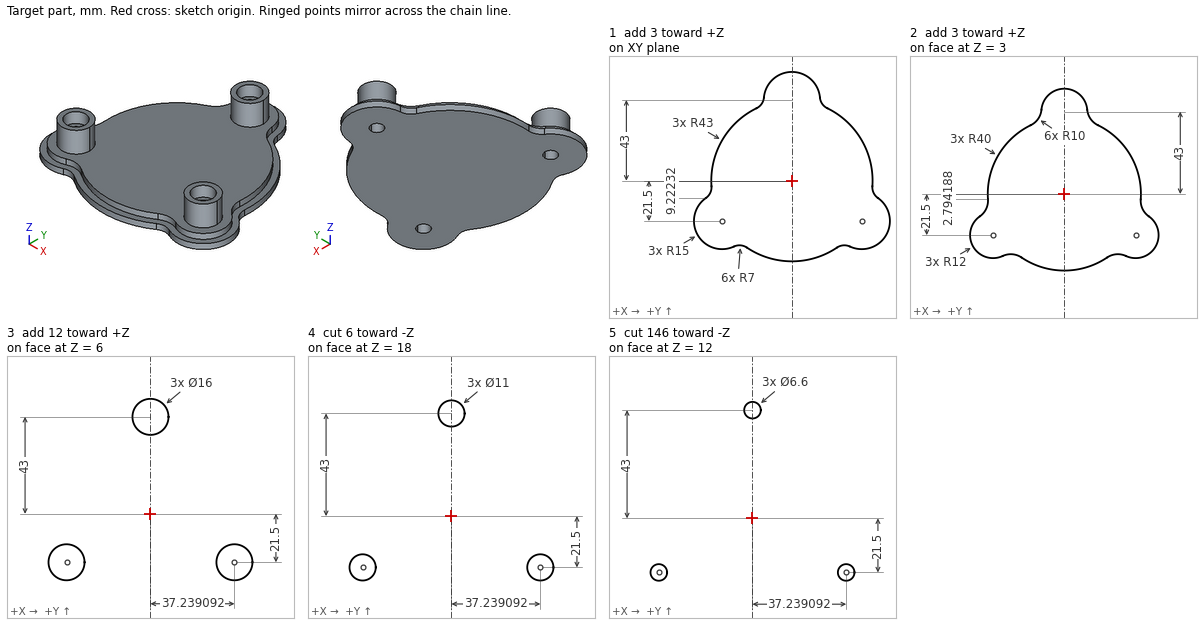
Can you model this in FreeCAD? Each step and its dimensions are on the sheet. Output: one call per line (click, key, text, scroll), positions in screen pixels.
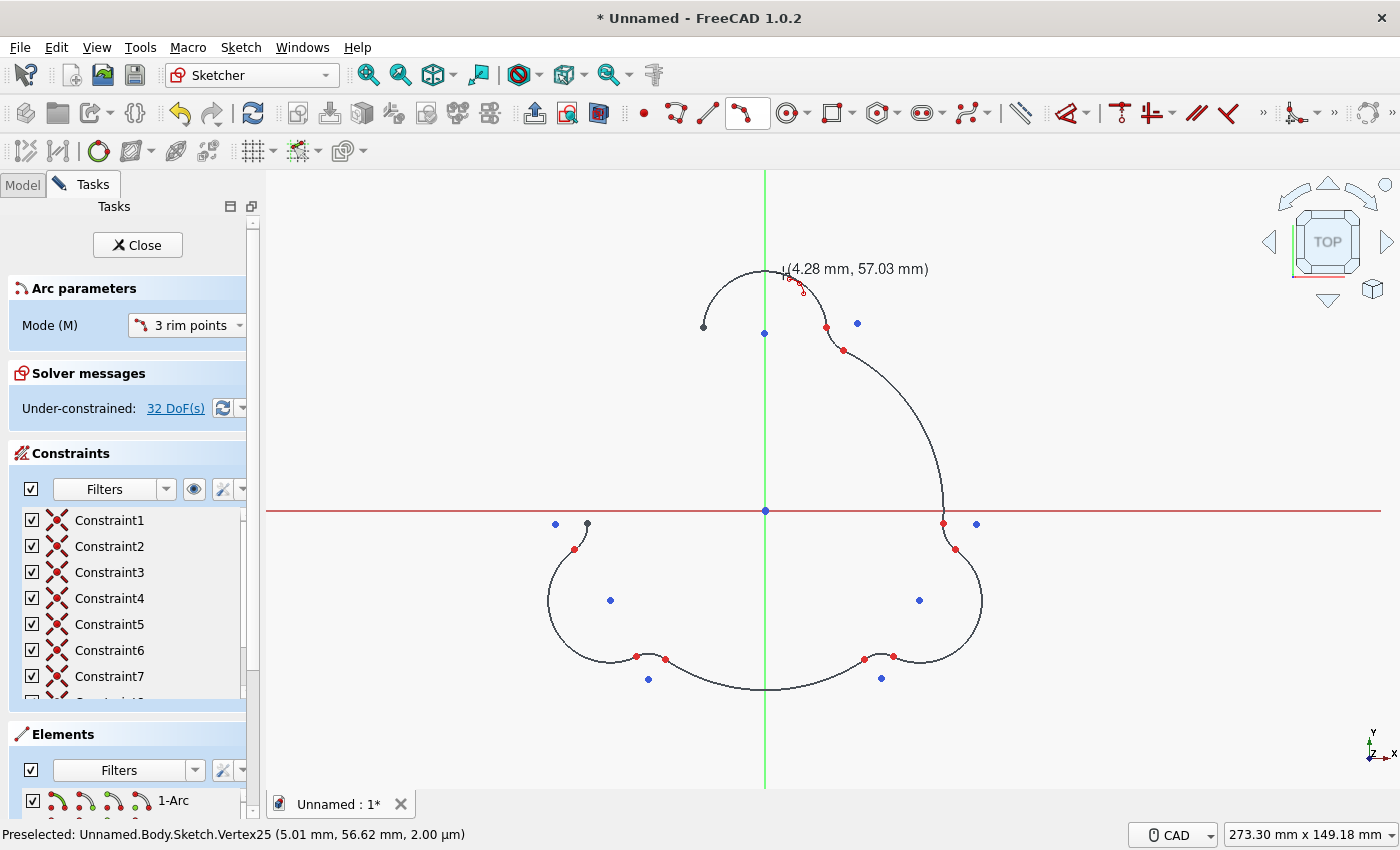
click(703, 328)
click(687, 350)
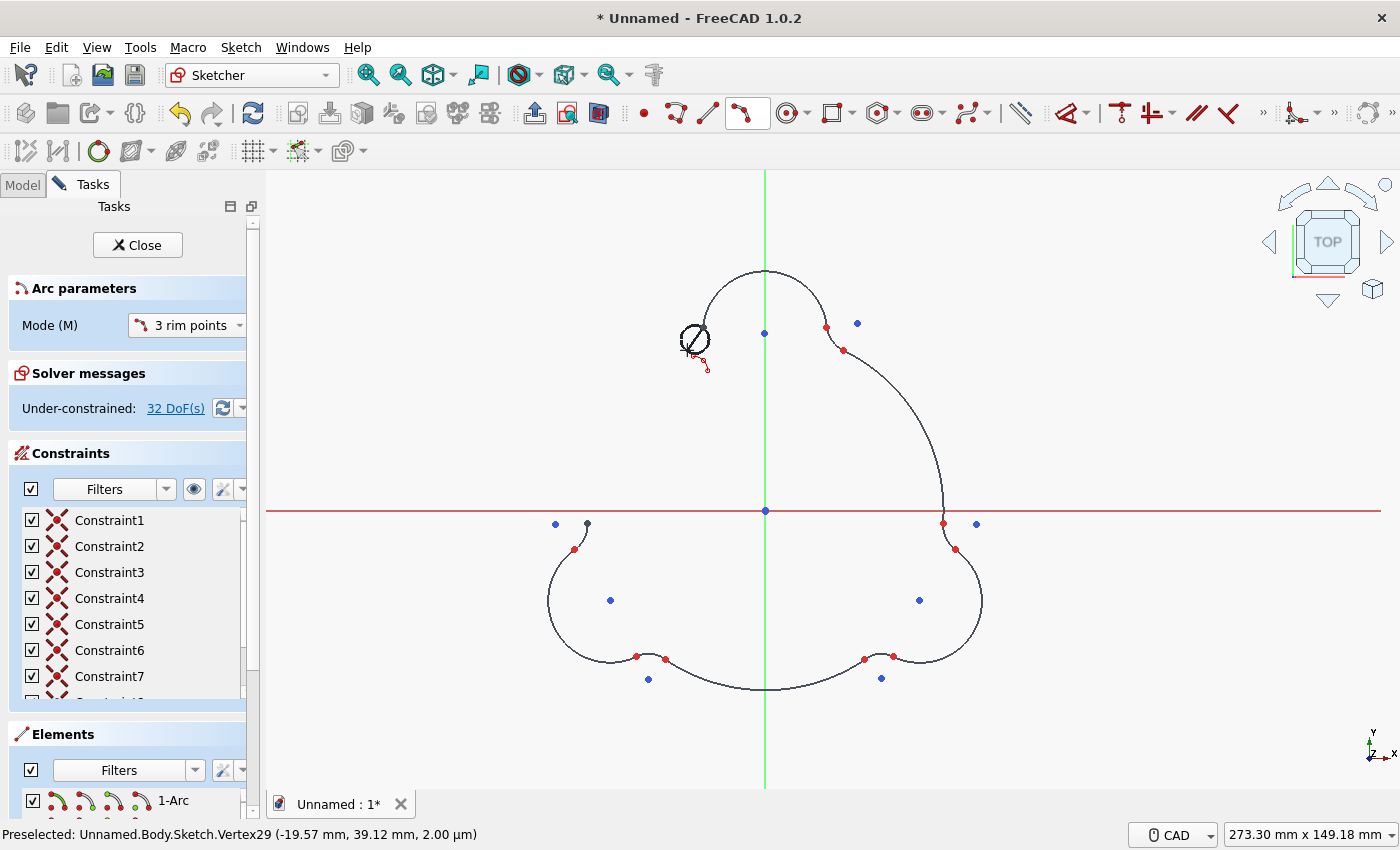
scroll(698, 341, up, 8)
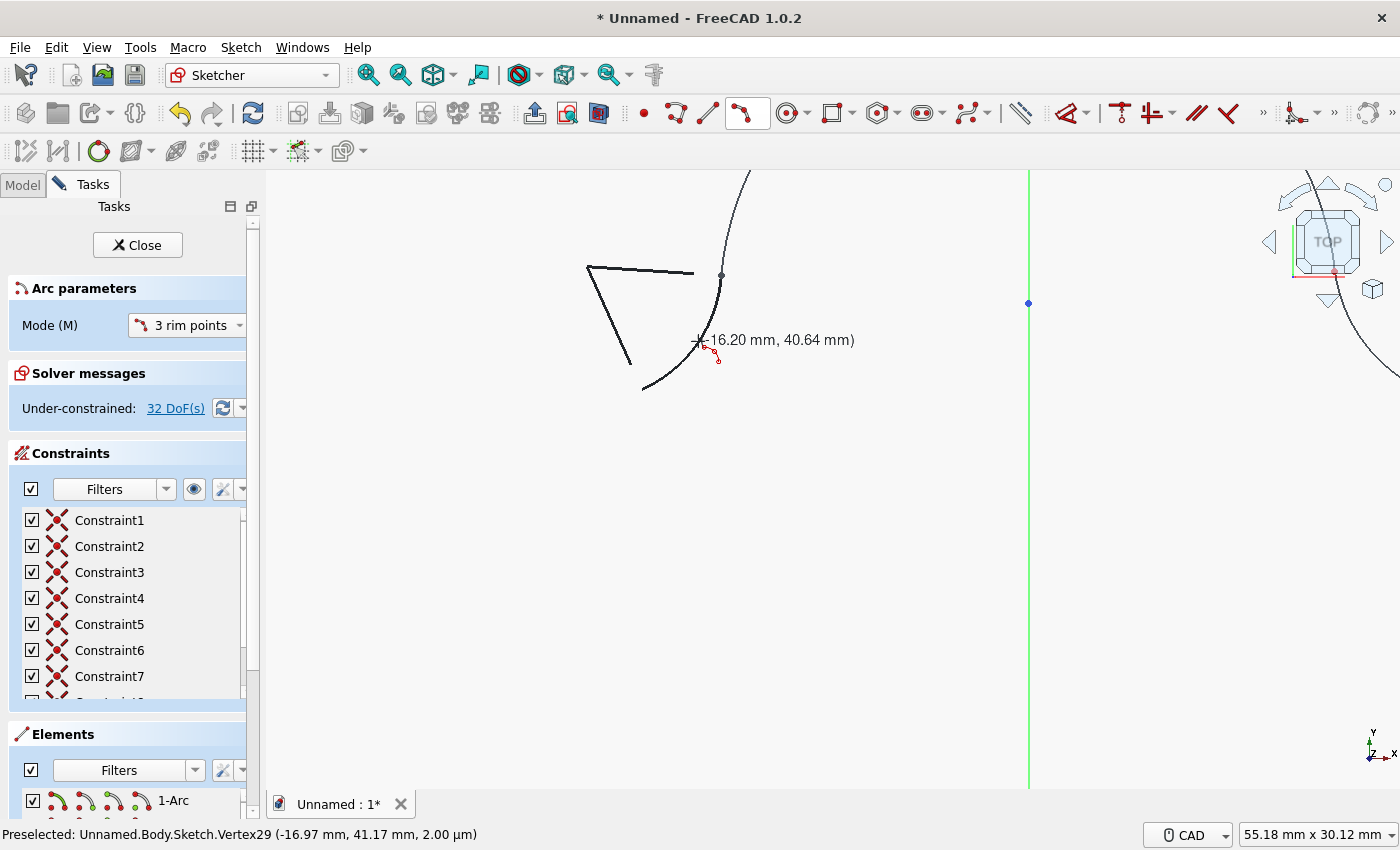
click(698, 338)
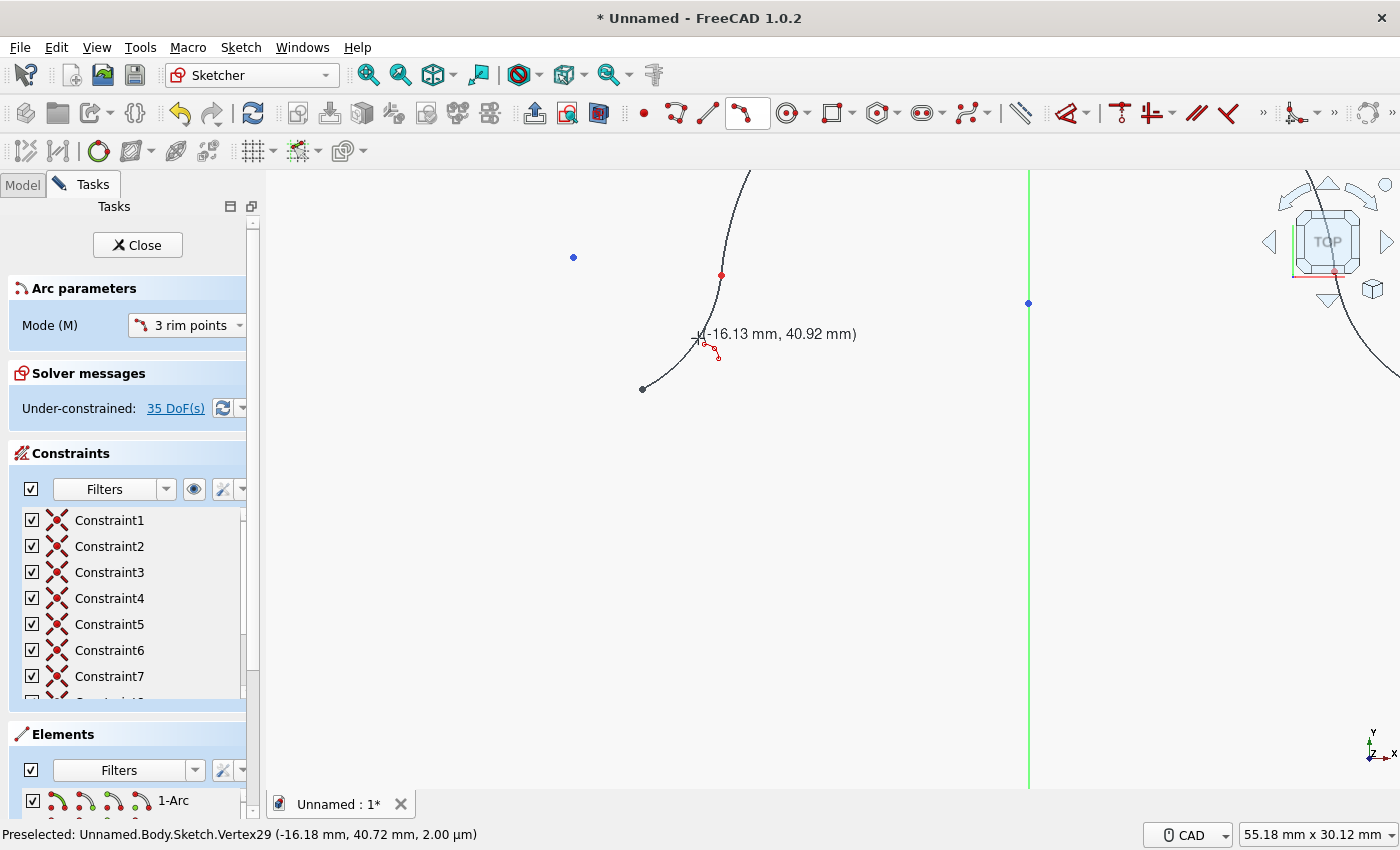
scroll(697, 341, down, 8)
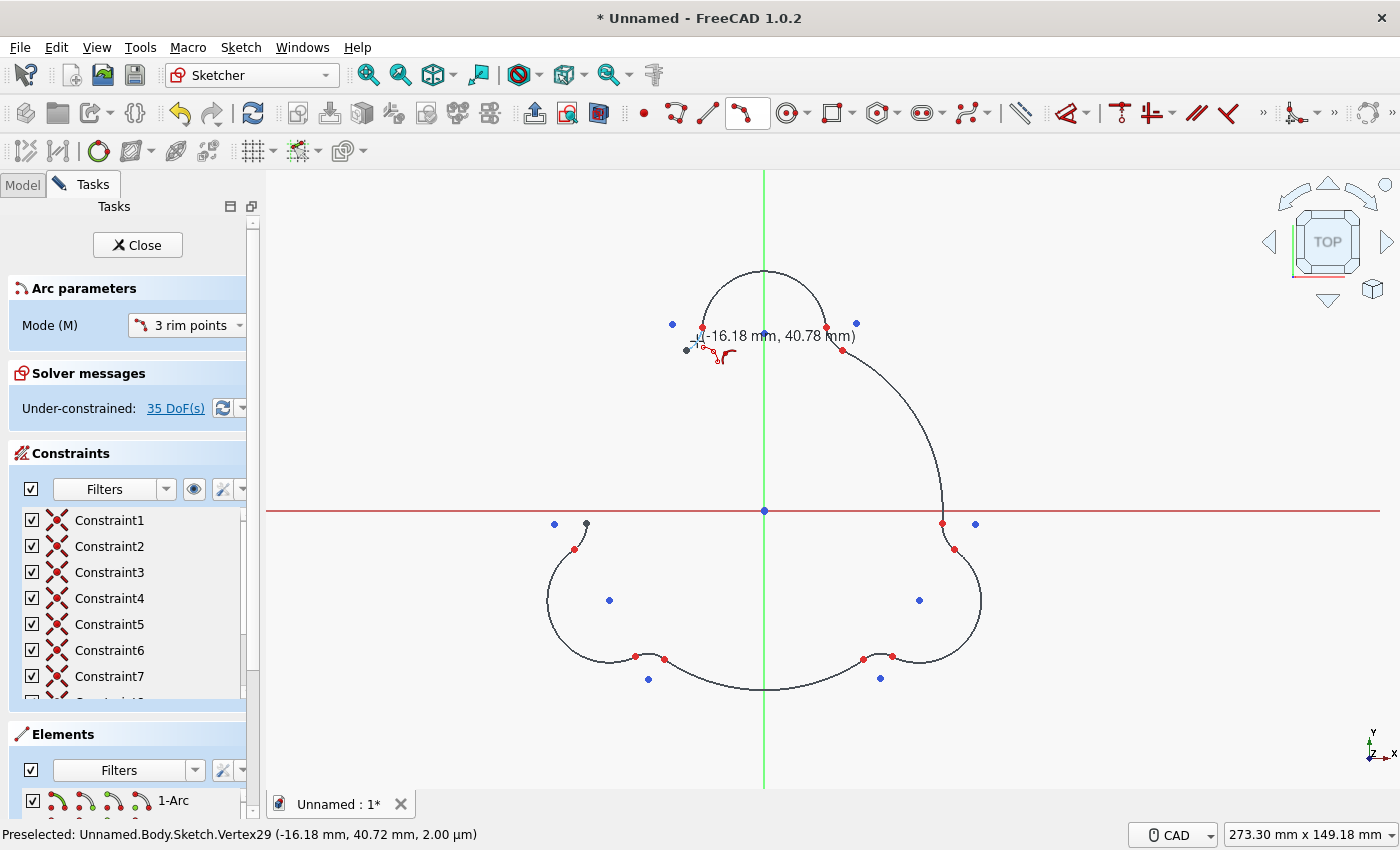
click(686, 351)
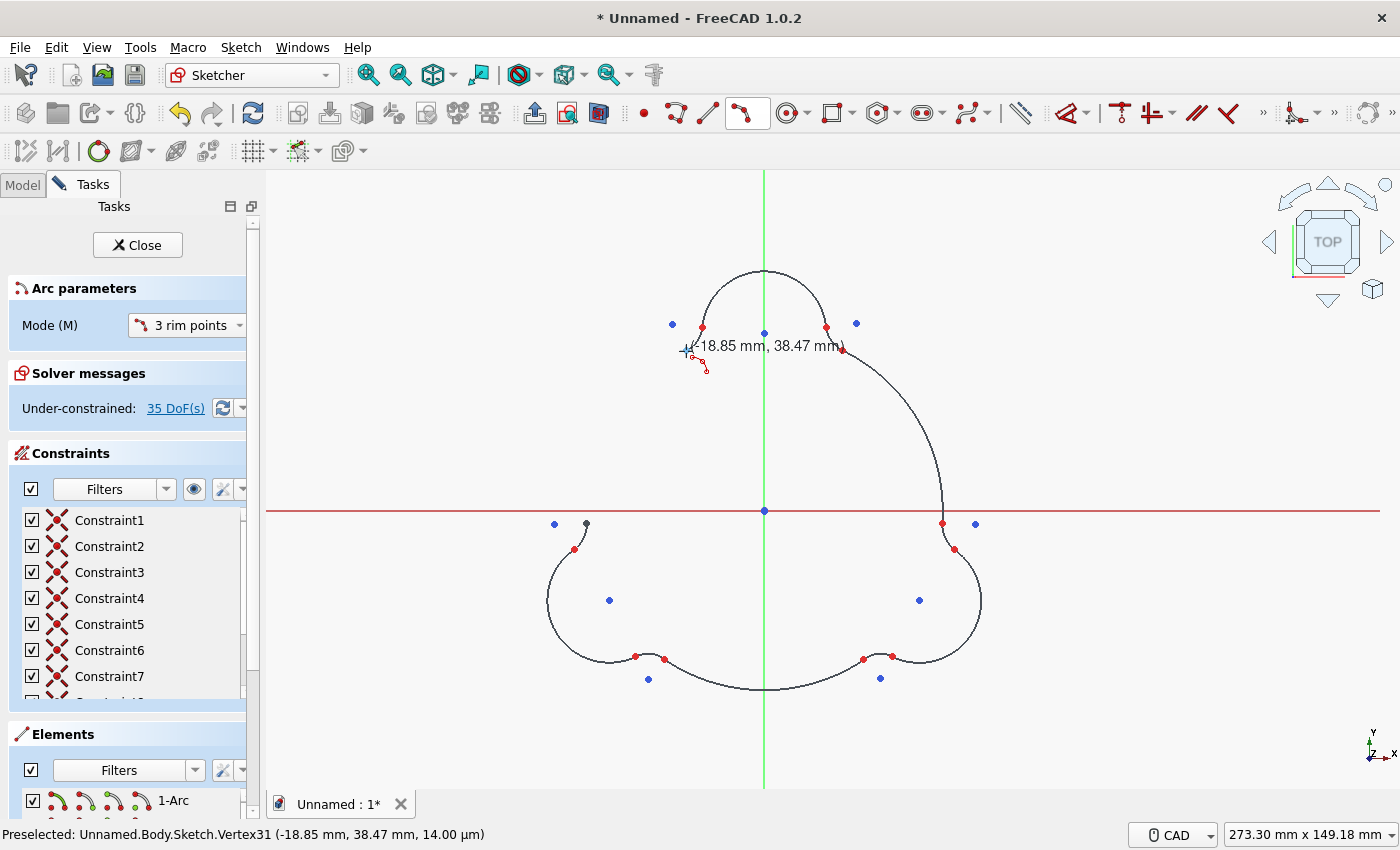
scroll(586, 523, up, 2)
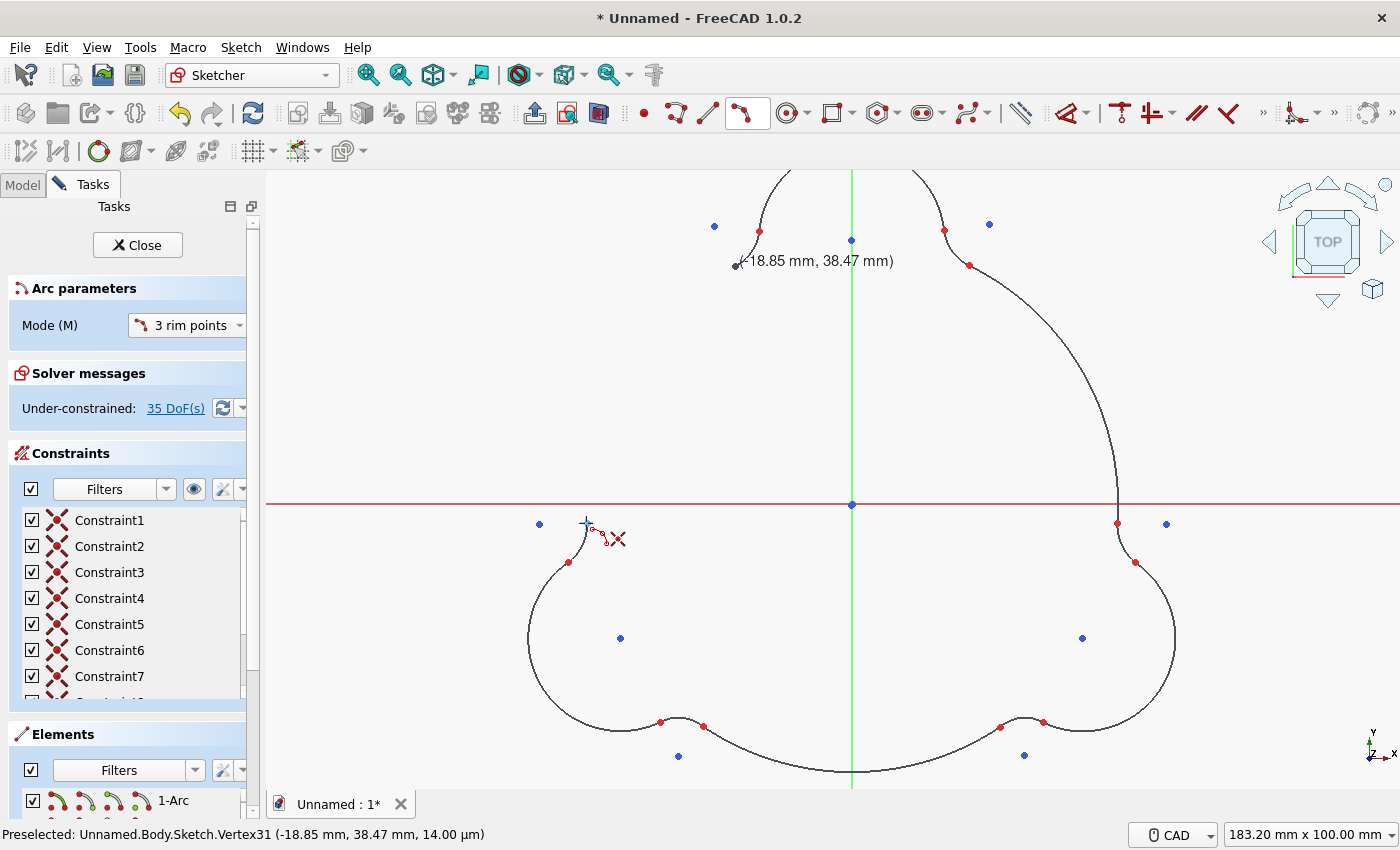
click(587, 524)
click(622, 371)
key(Escape)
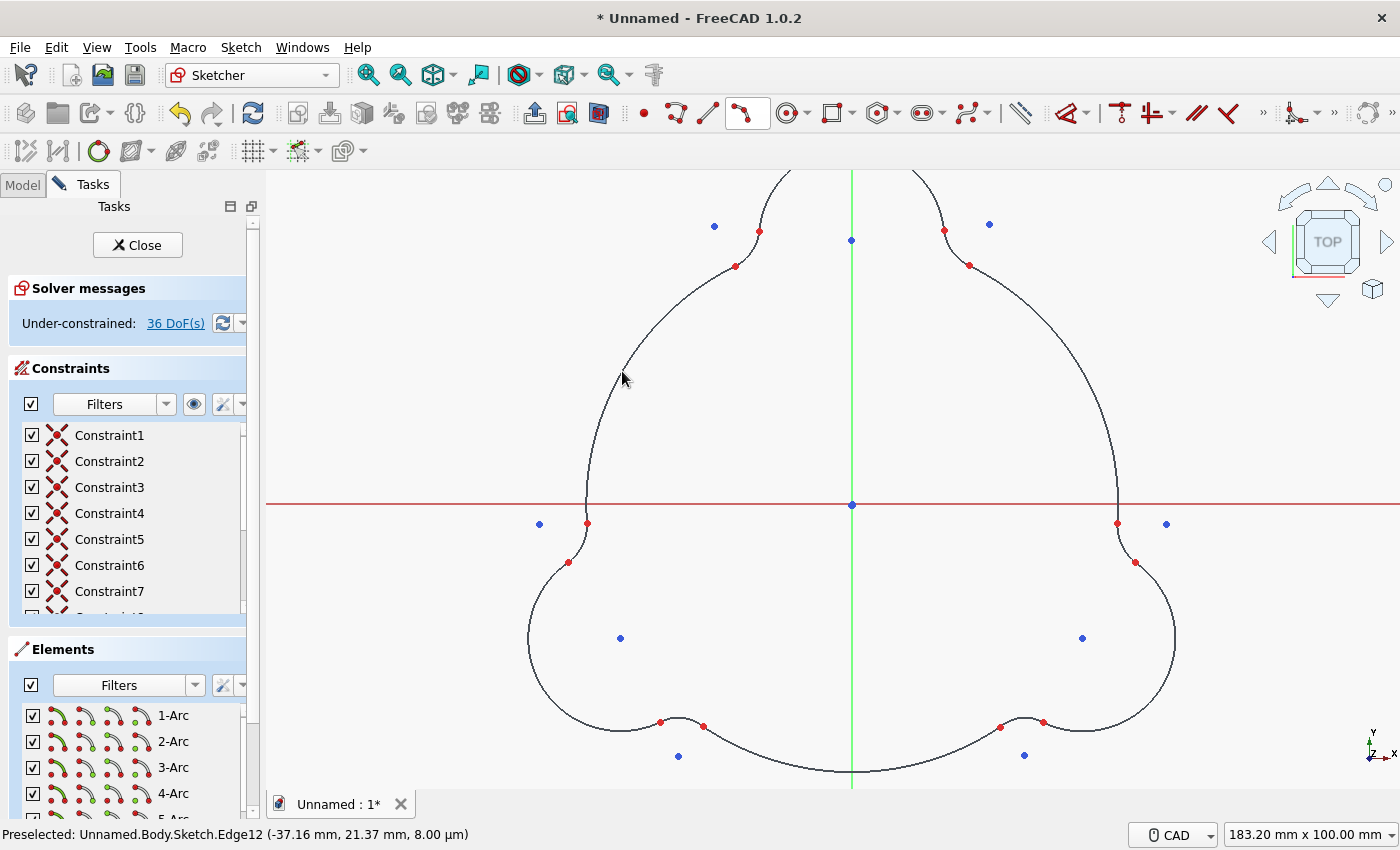
click(578, 553)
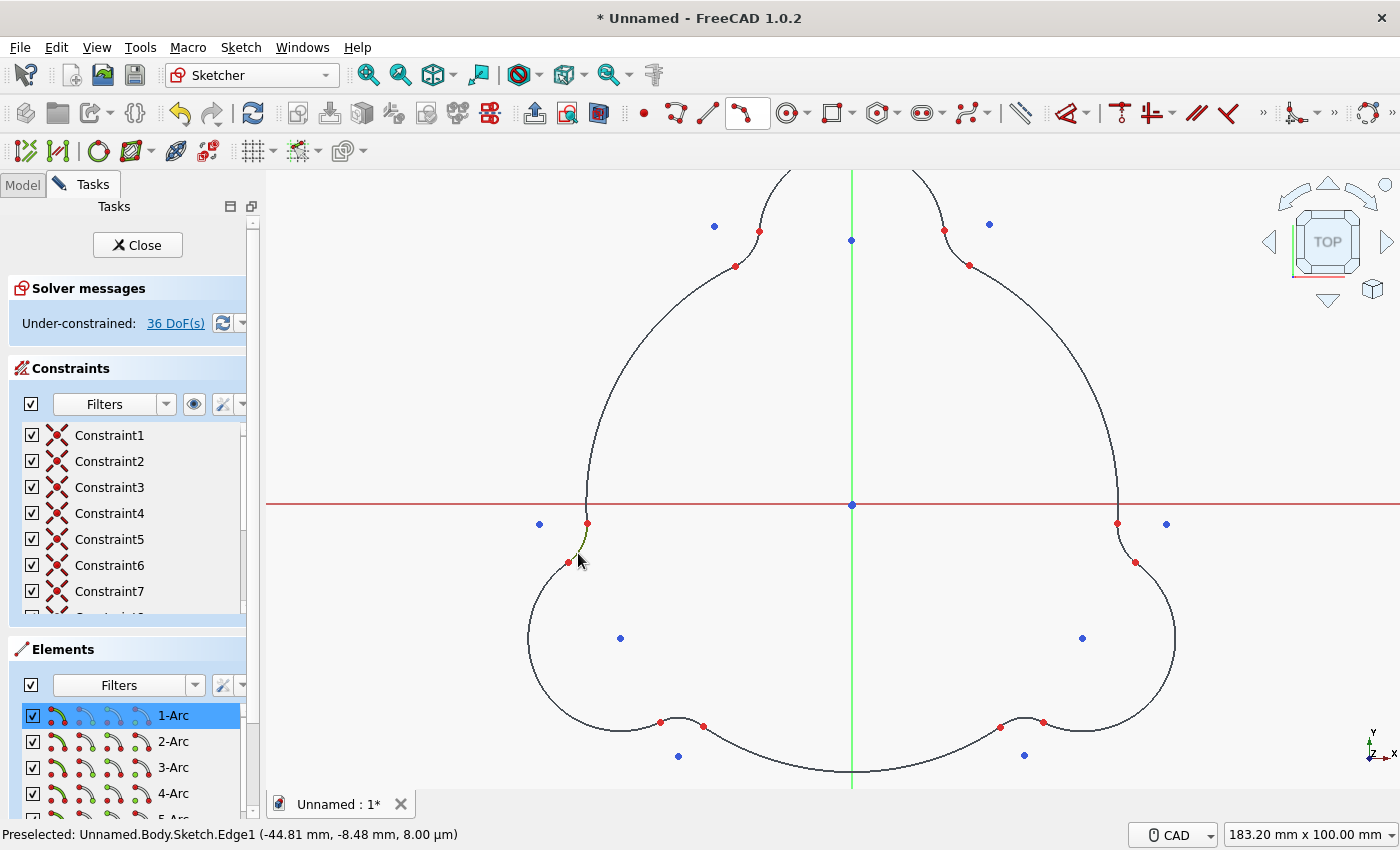
click(529, 632)